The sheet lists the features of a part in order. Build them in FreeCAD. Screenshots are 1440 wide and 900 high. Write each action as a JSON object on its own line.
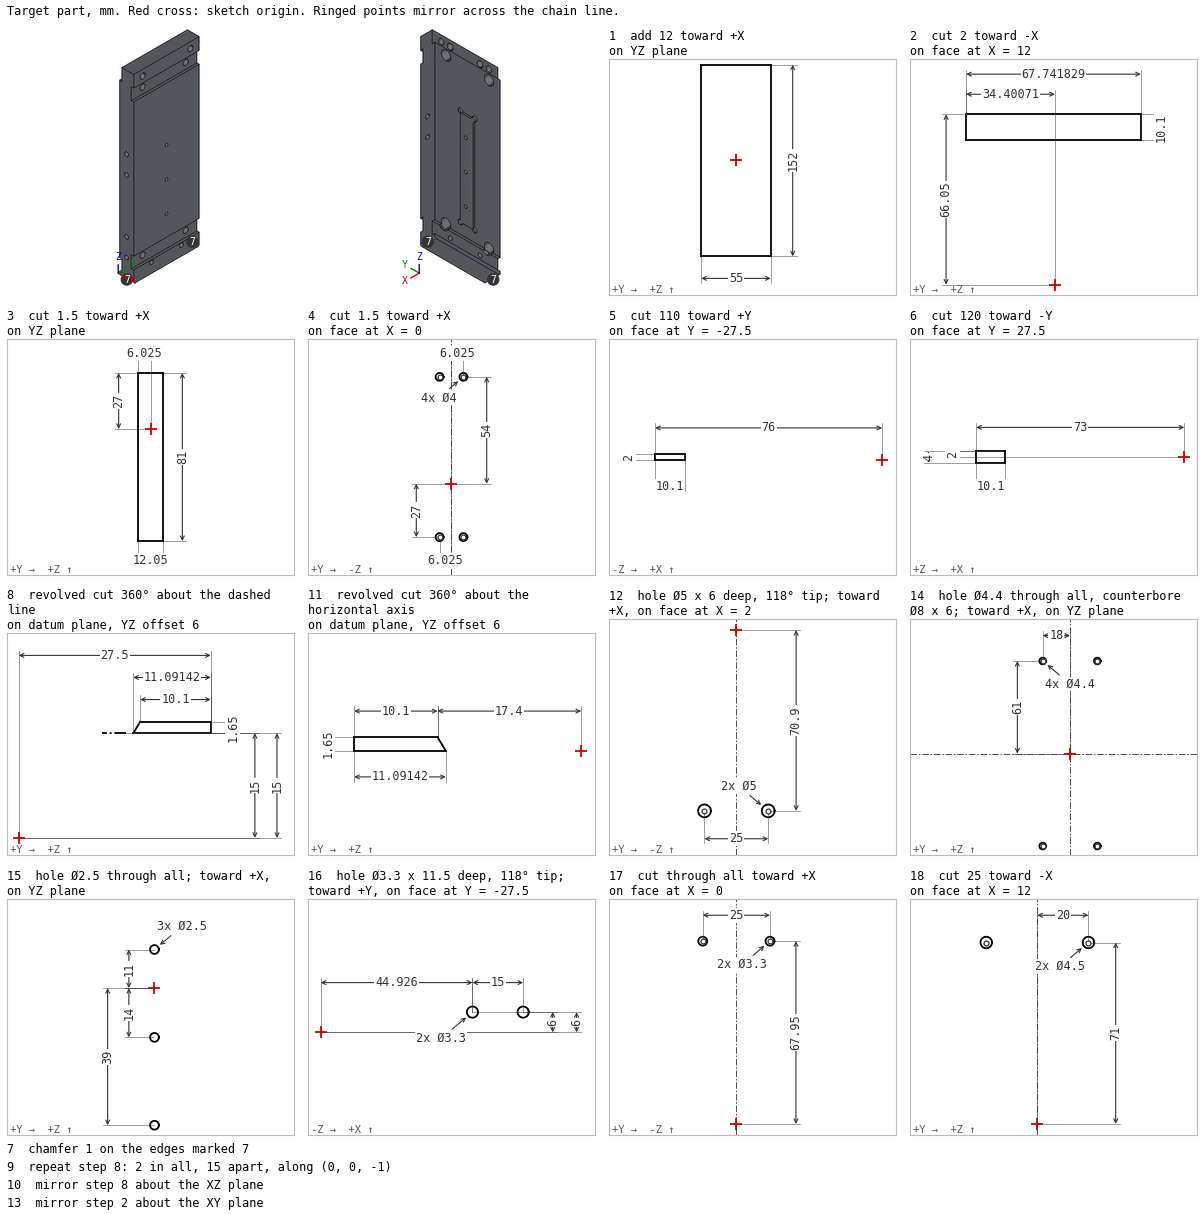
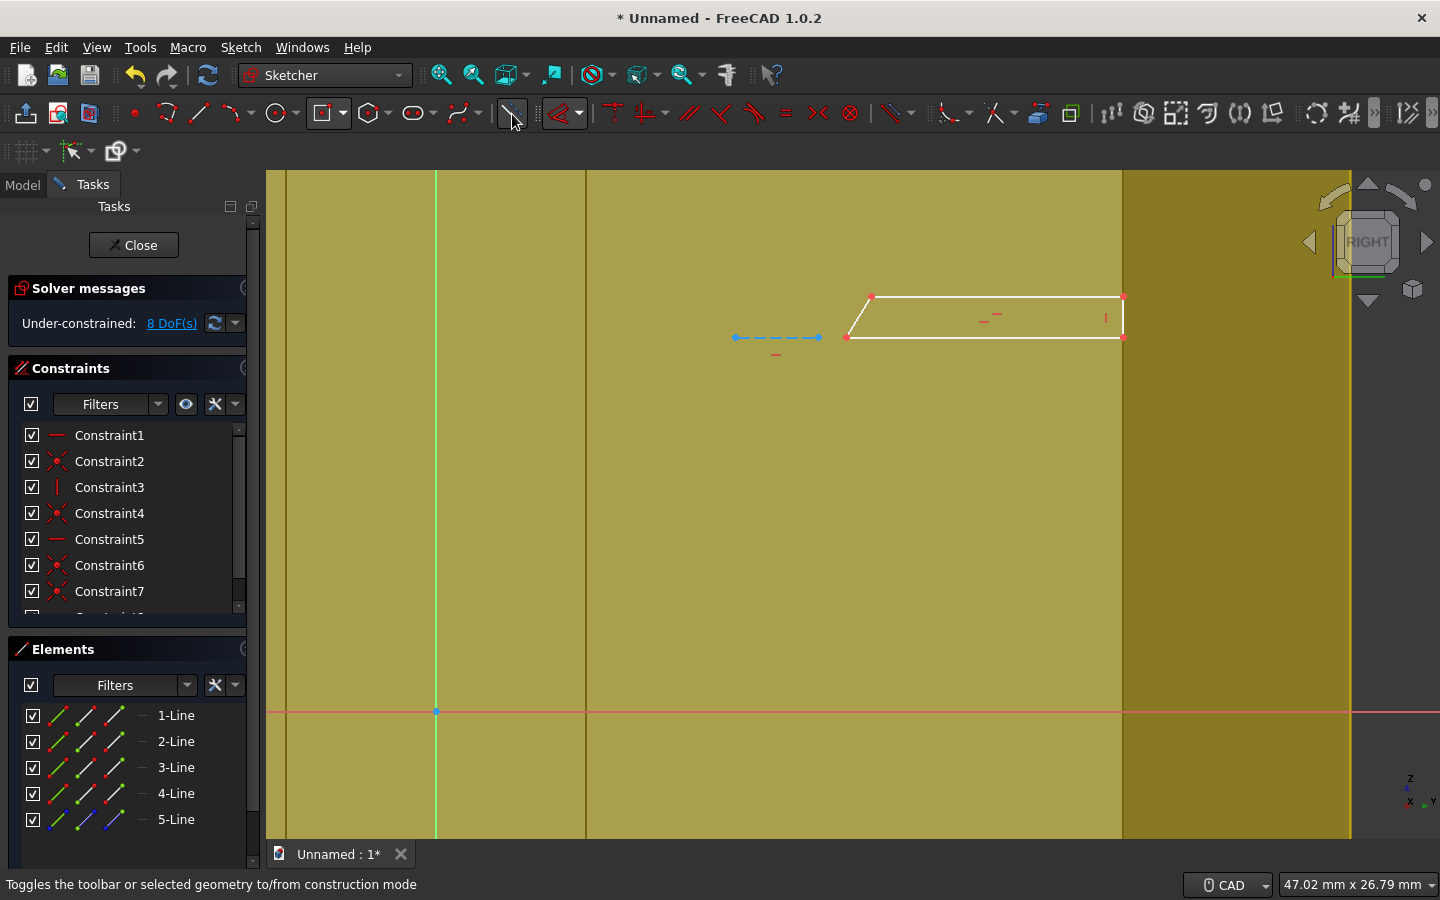
{"action": "left_click", "coordinate": [846, 338]}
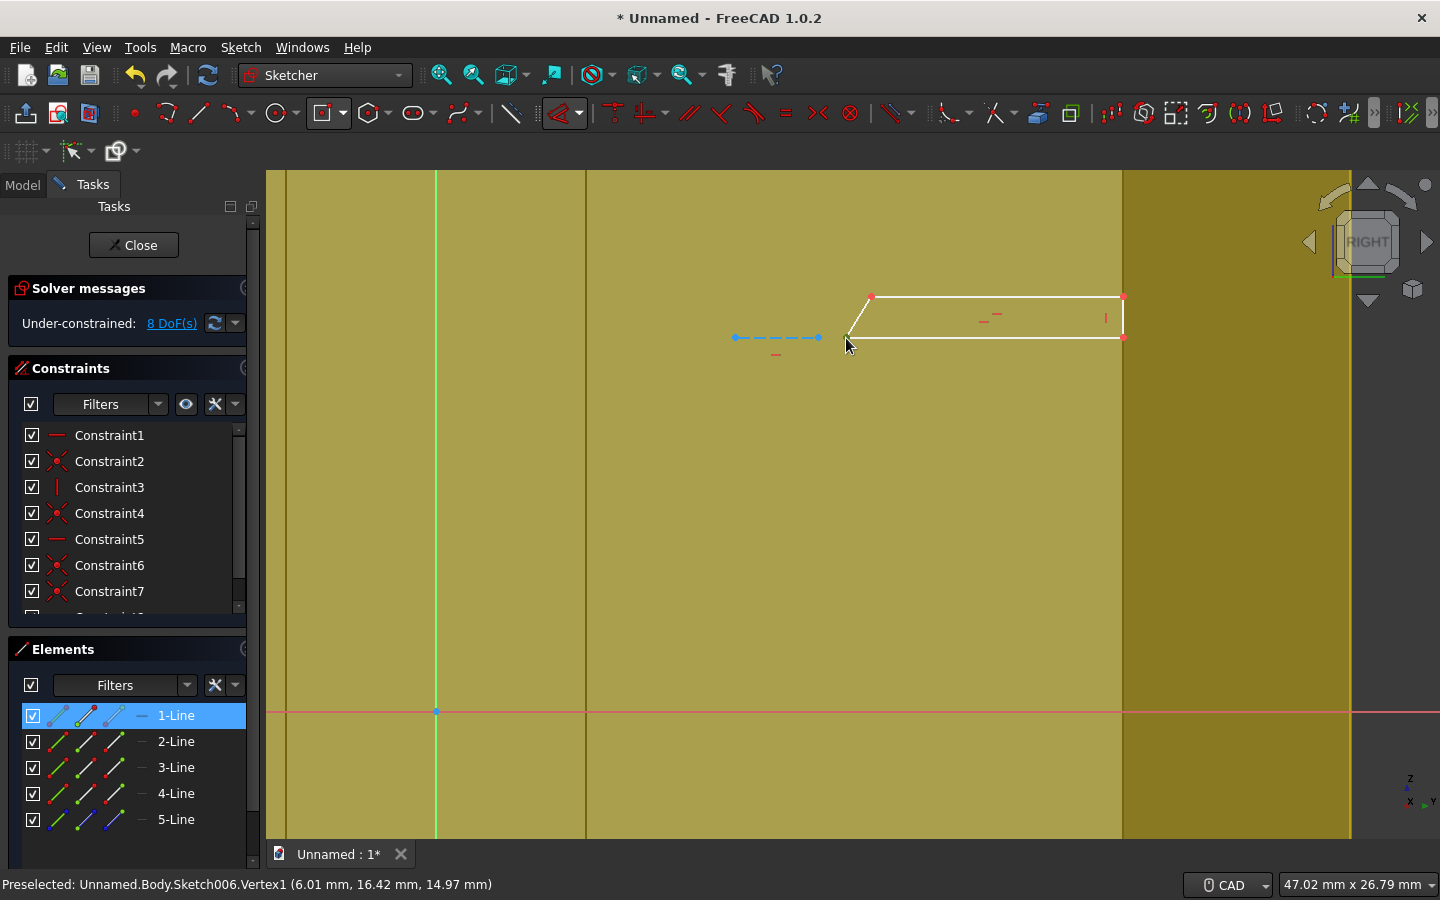
{"action": "key", "text": "i"}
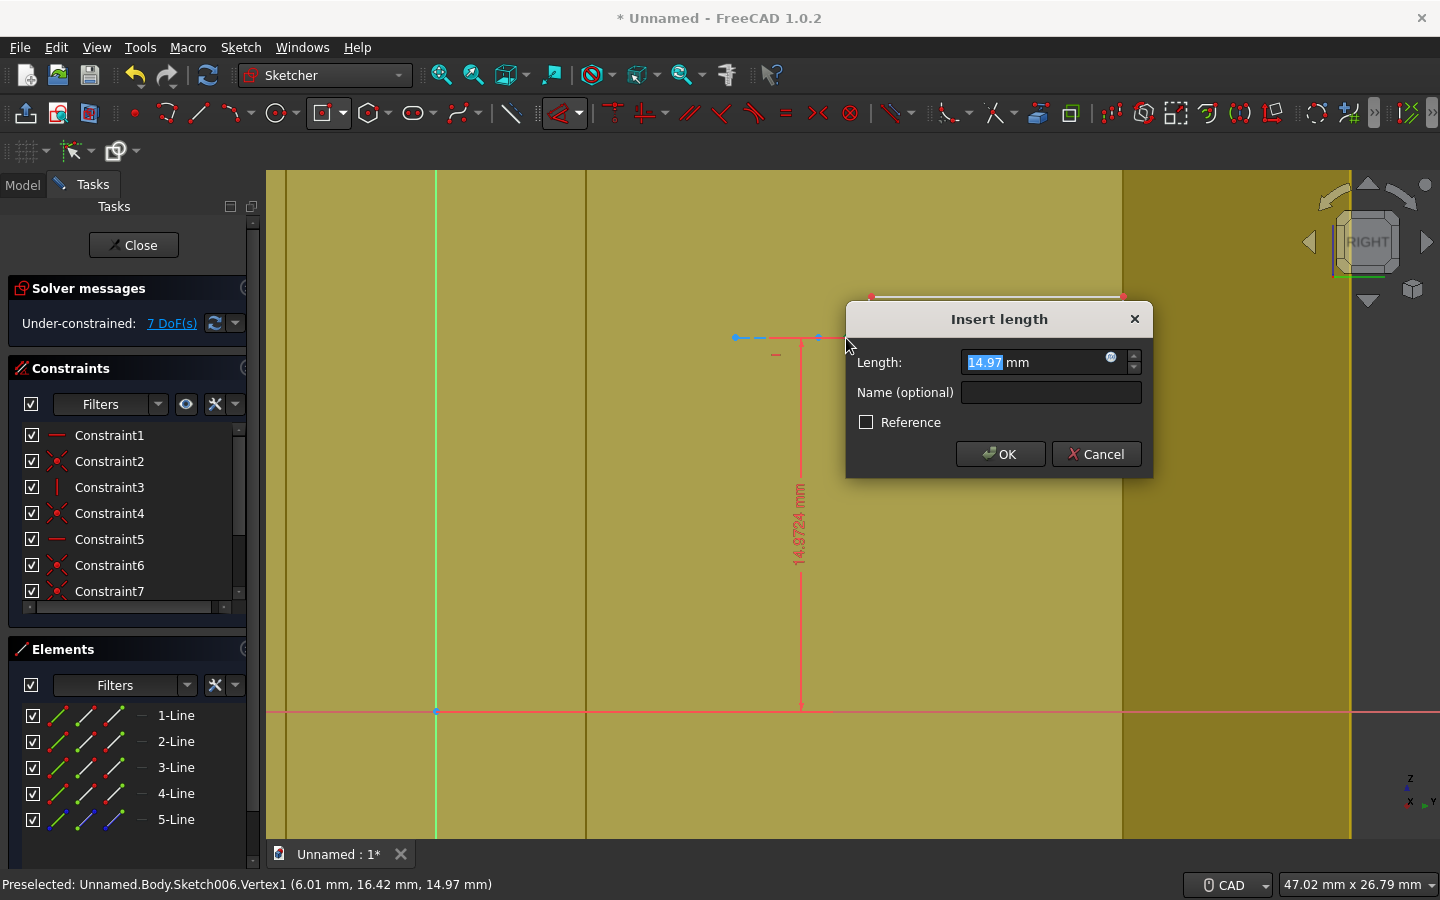
{"action": "type", "text": "15"}
{"action": "key", "text": "Return"}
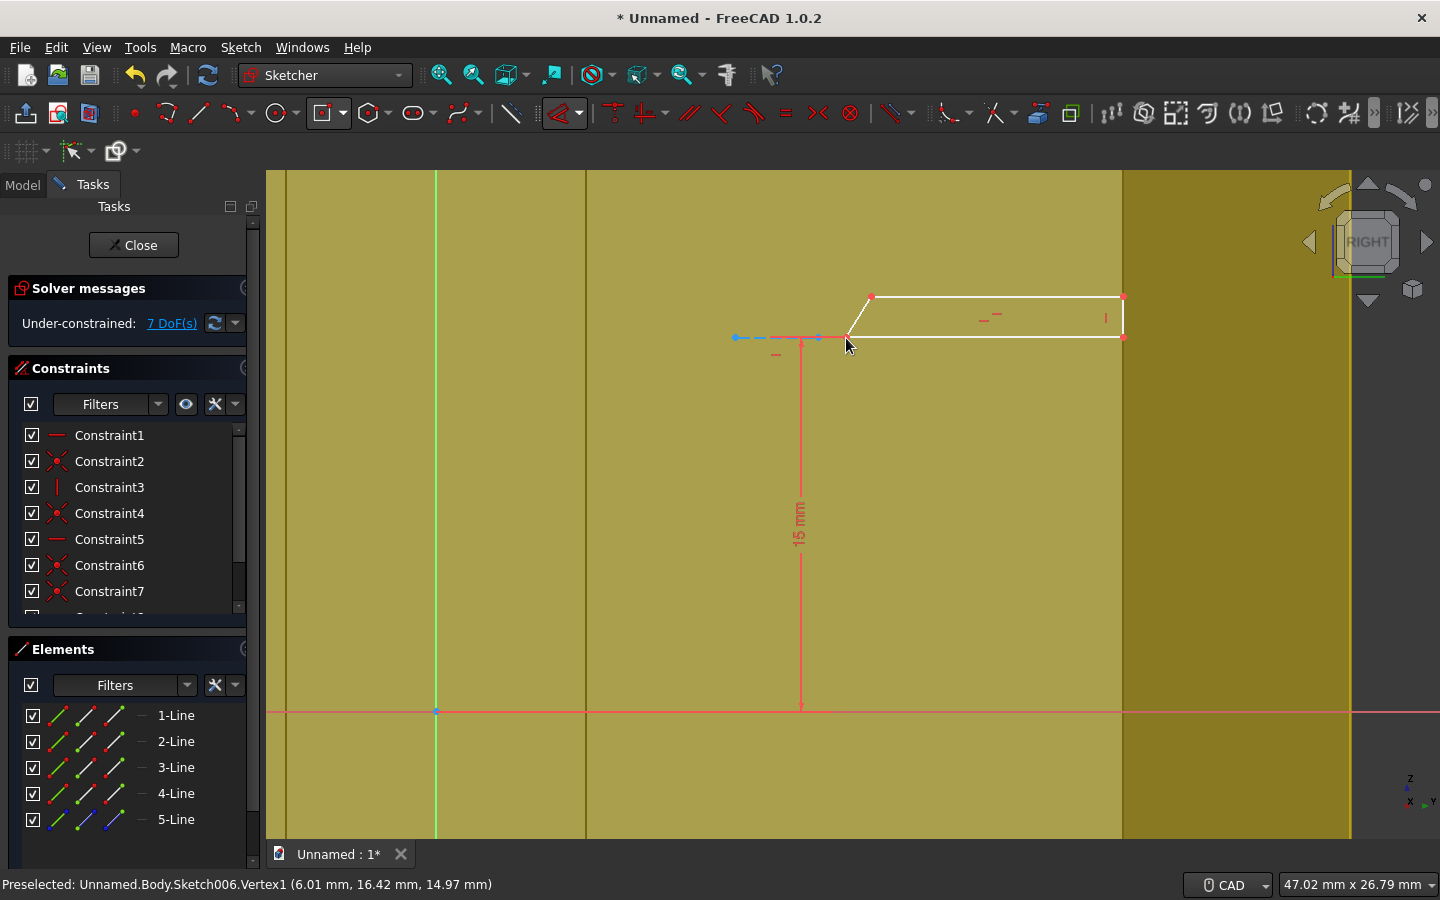
{"action": "left_click", "coordinate": [818, 338]}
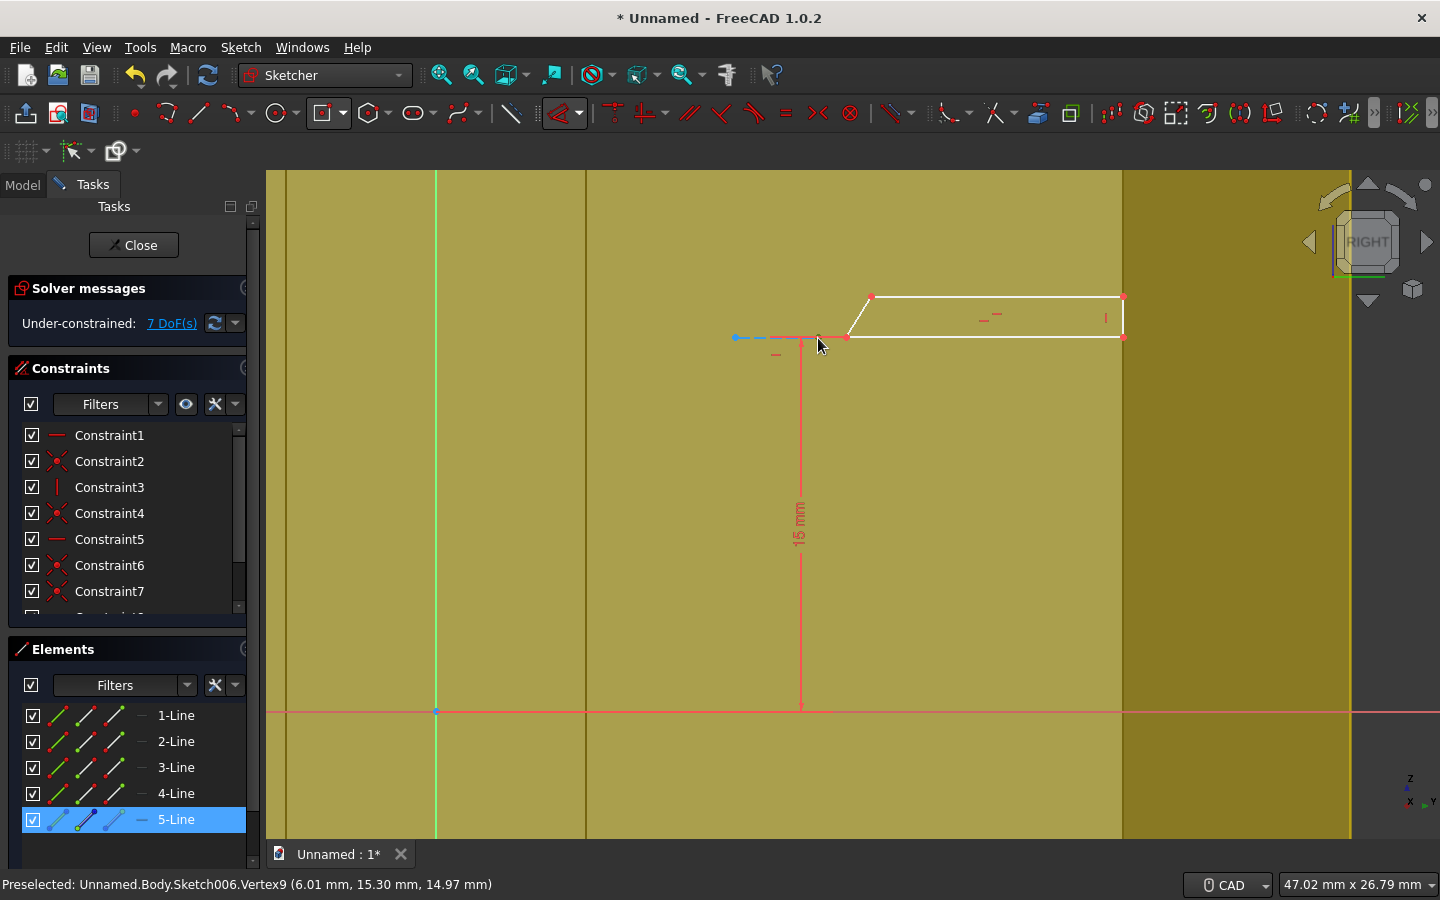
{"action": "key", "text": "i"}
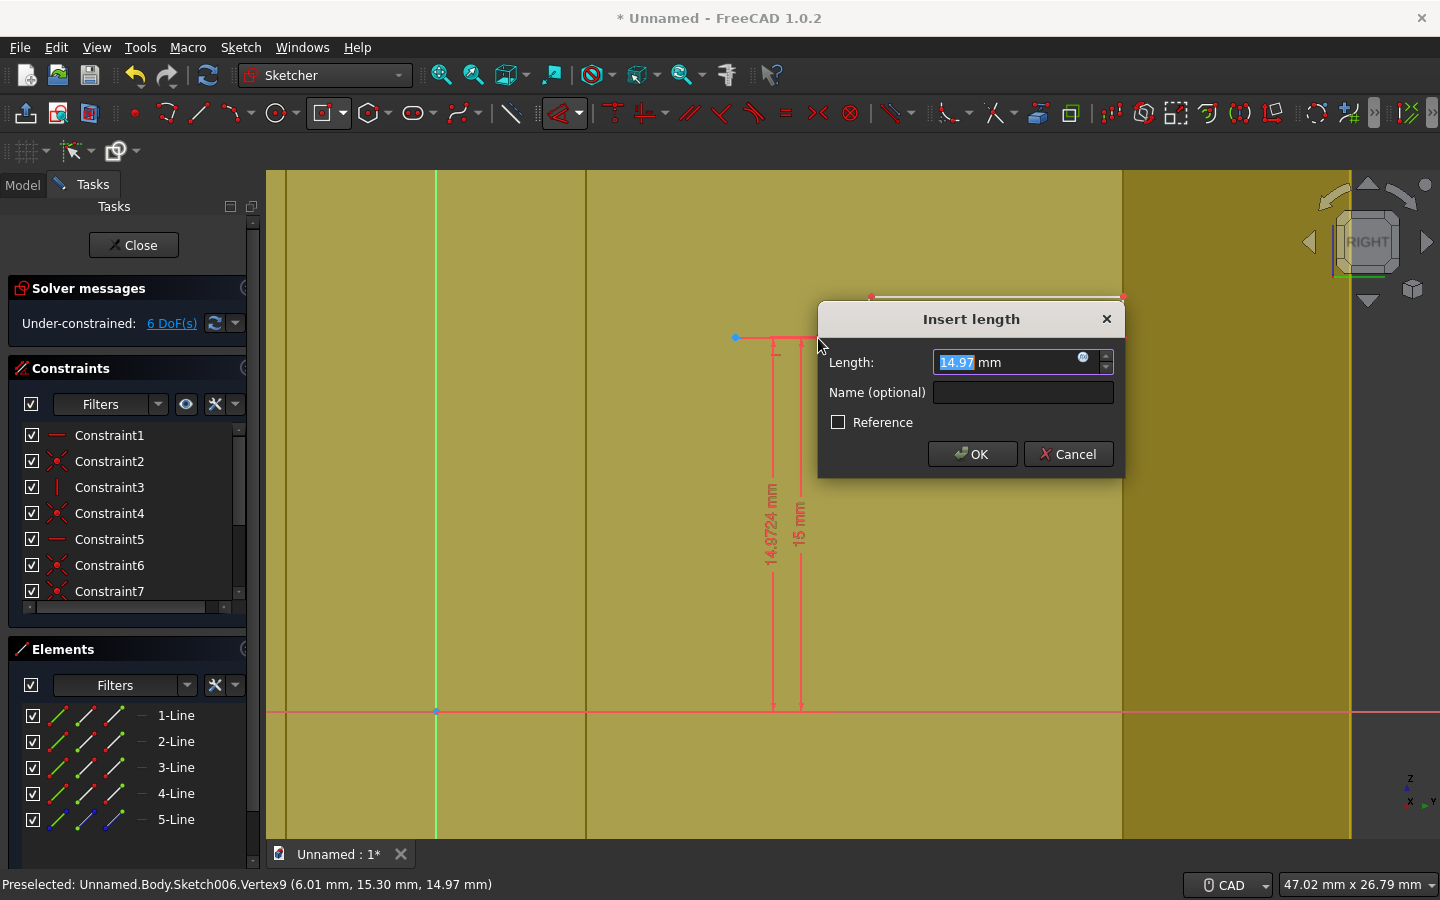
{"action": "type", "text": "15"}
{"action": "key", "text": "Return"}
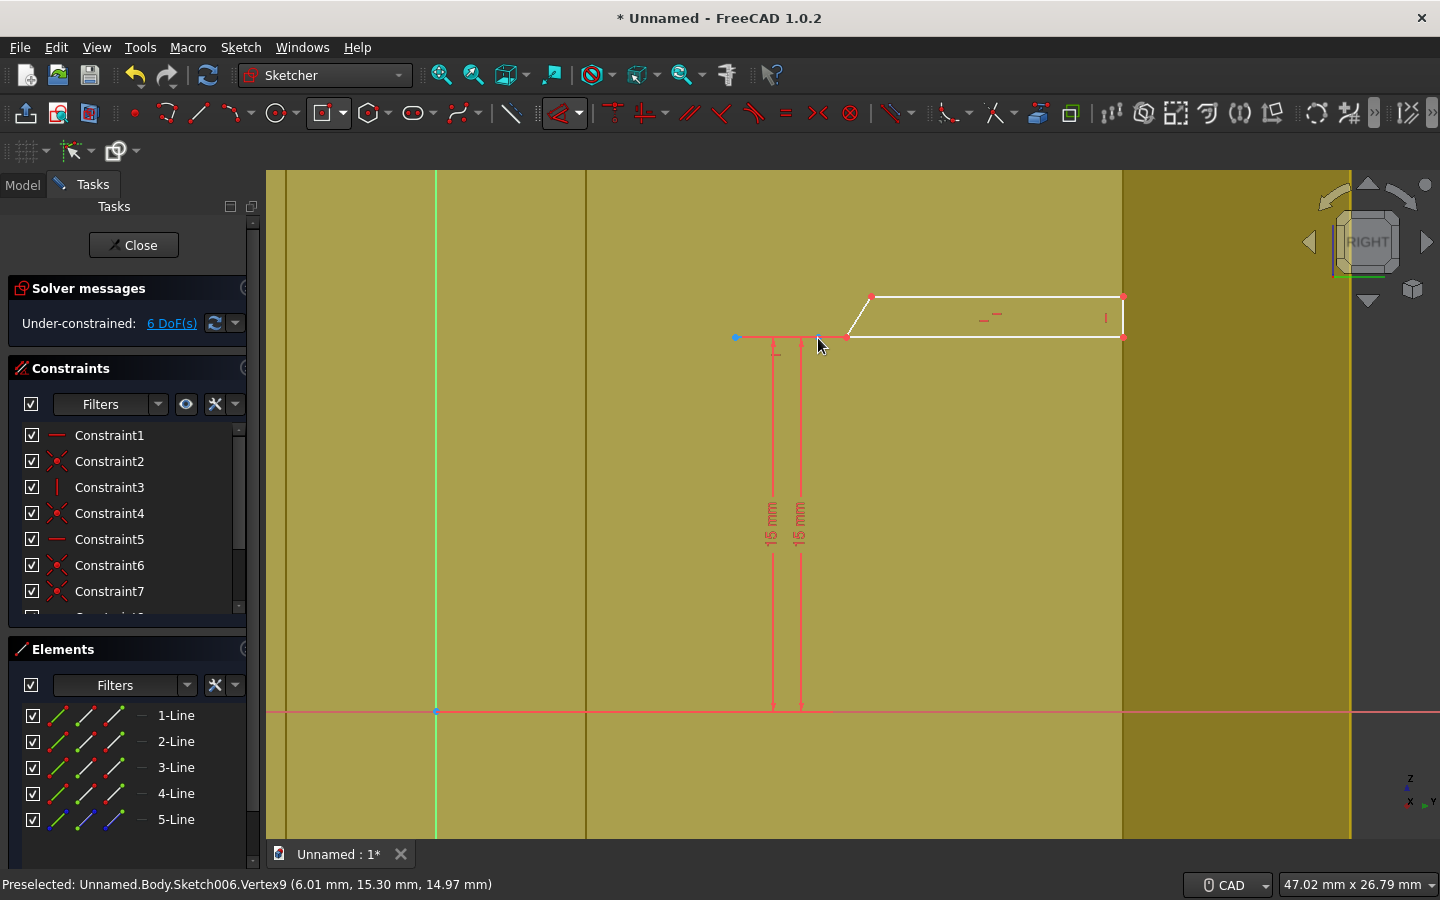
{"action": "left_click", "coordinate": [1123, 325]}